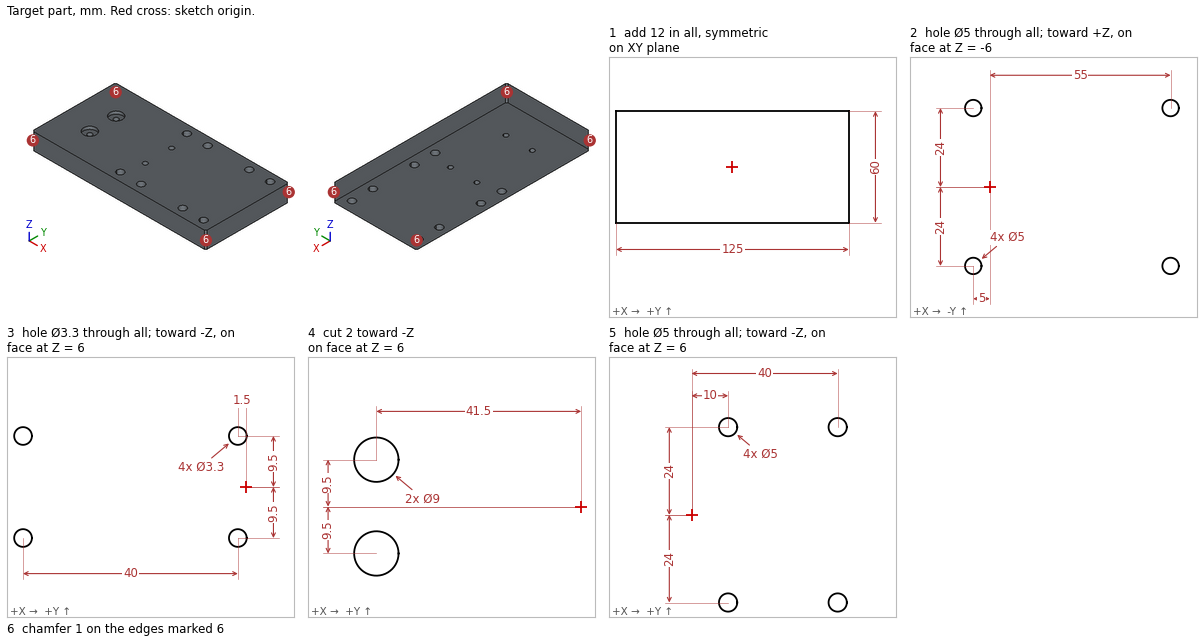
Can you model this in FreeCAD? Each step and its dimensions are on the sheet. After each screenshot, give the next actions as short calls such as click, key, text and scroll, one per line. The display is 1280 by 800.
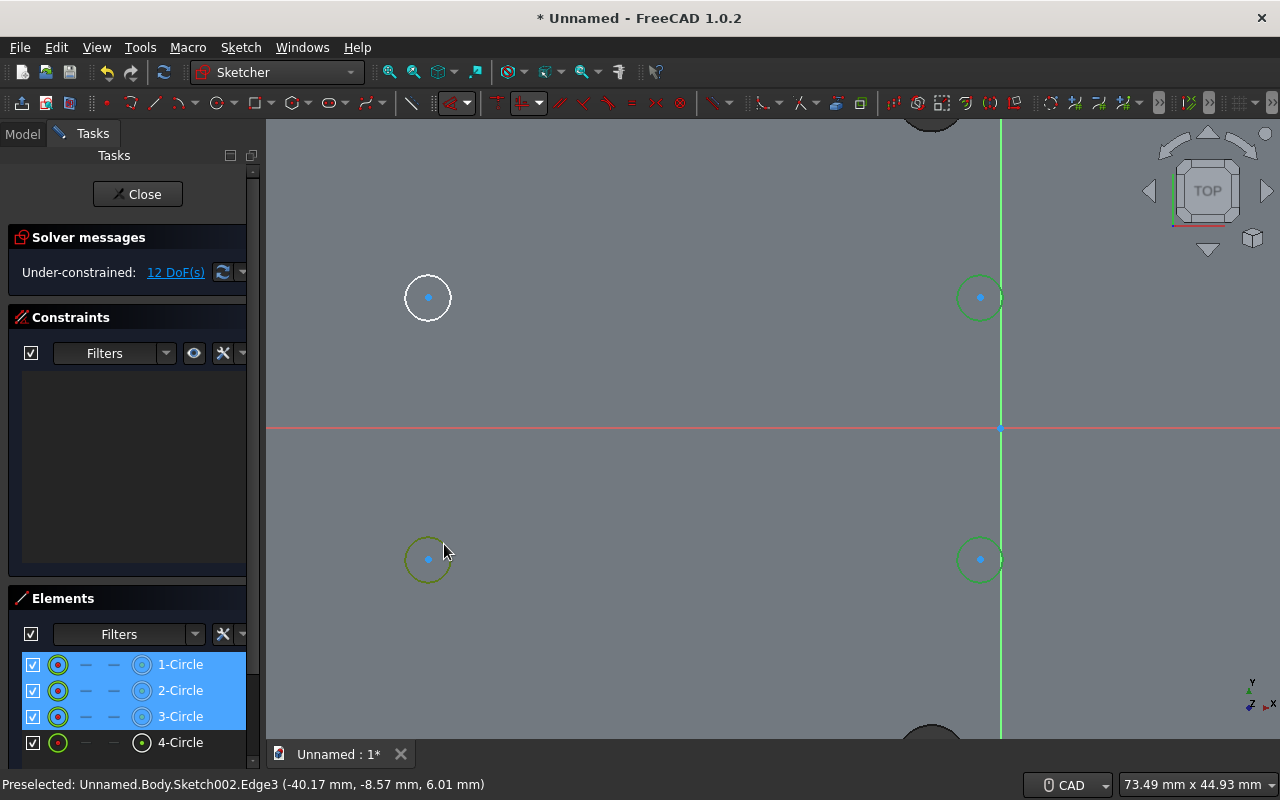
click(444, 282)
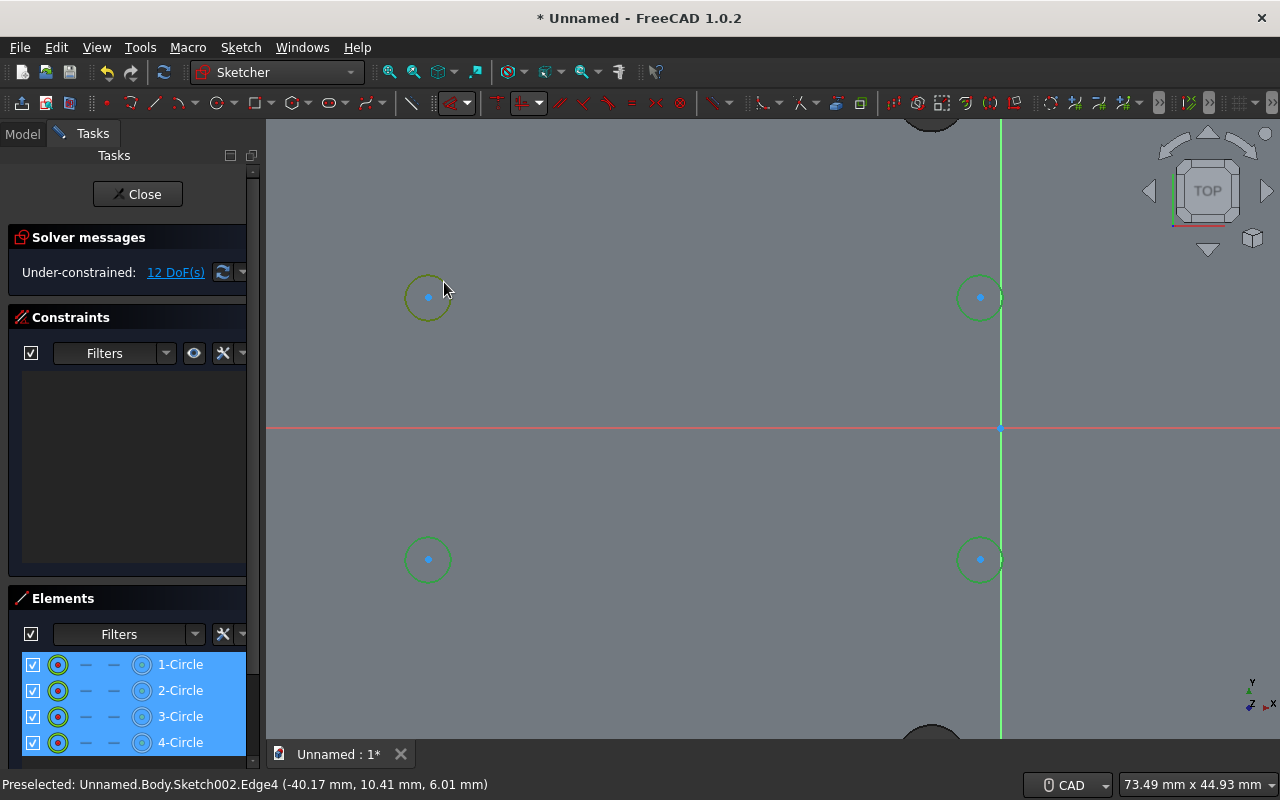
key(e)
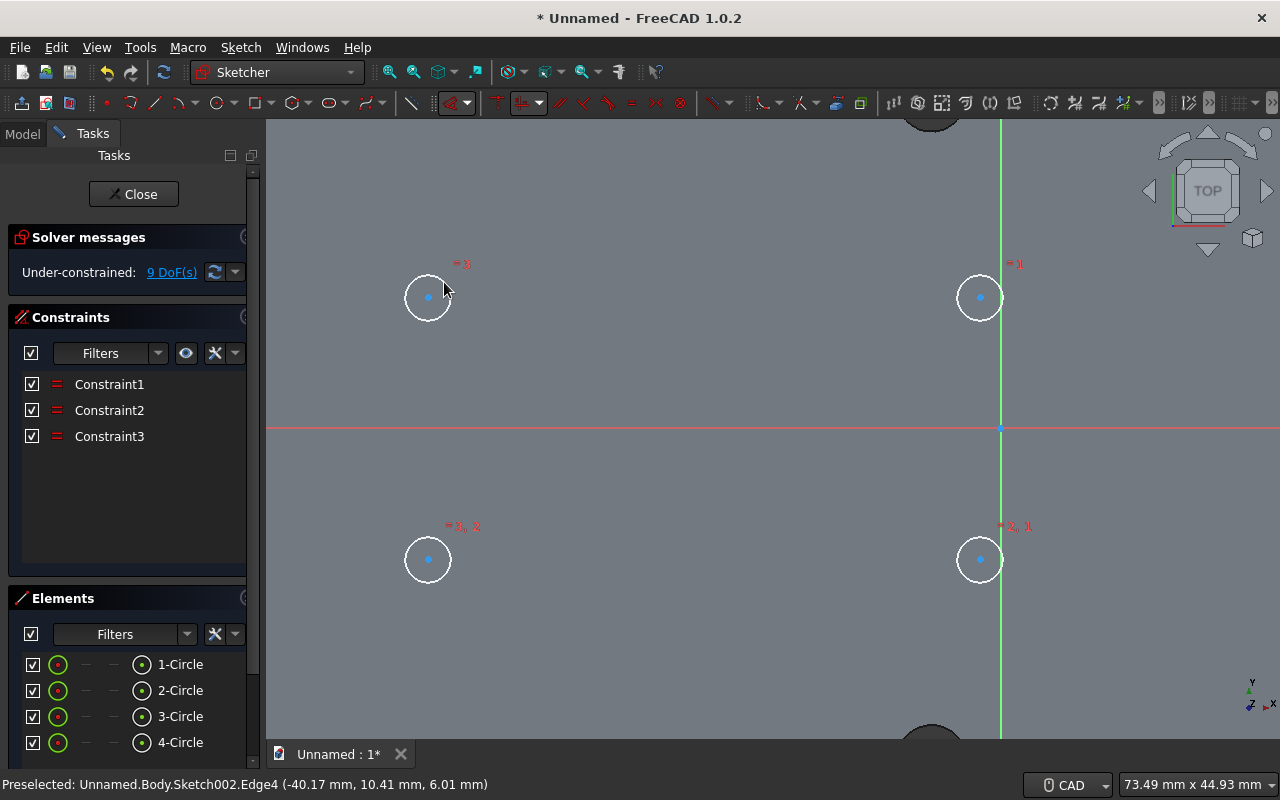
click(980, 298)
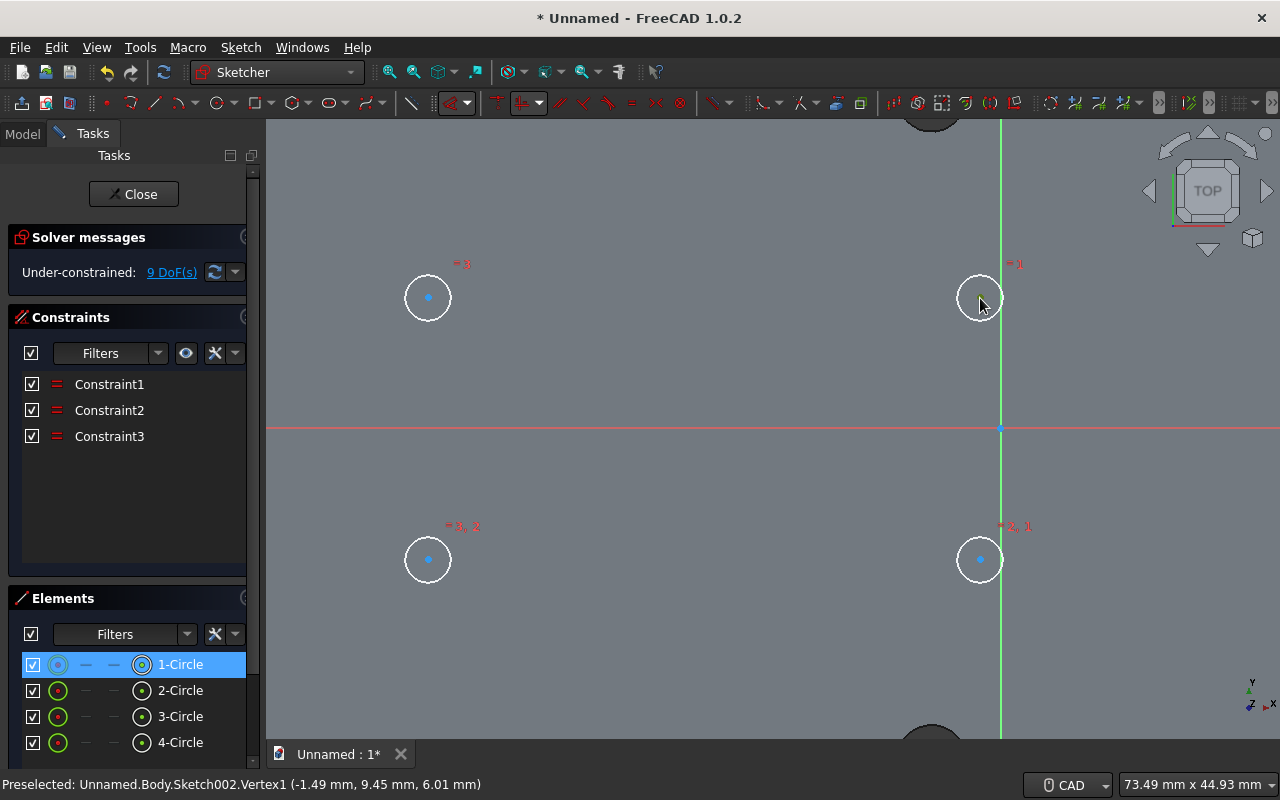
click(980, 560)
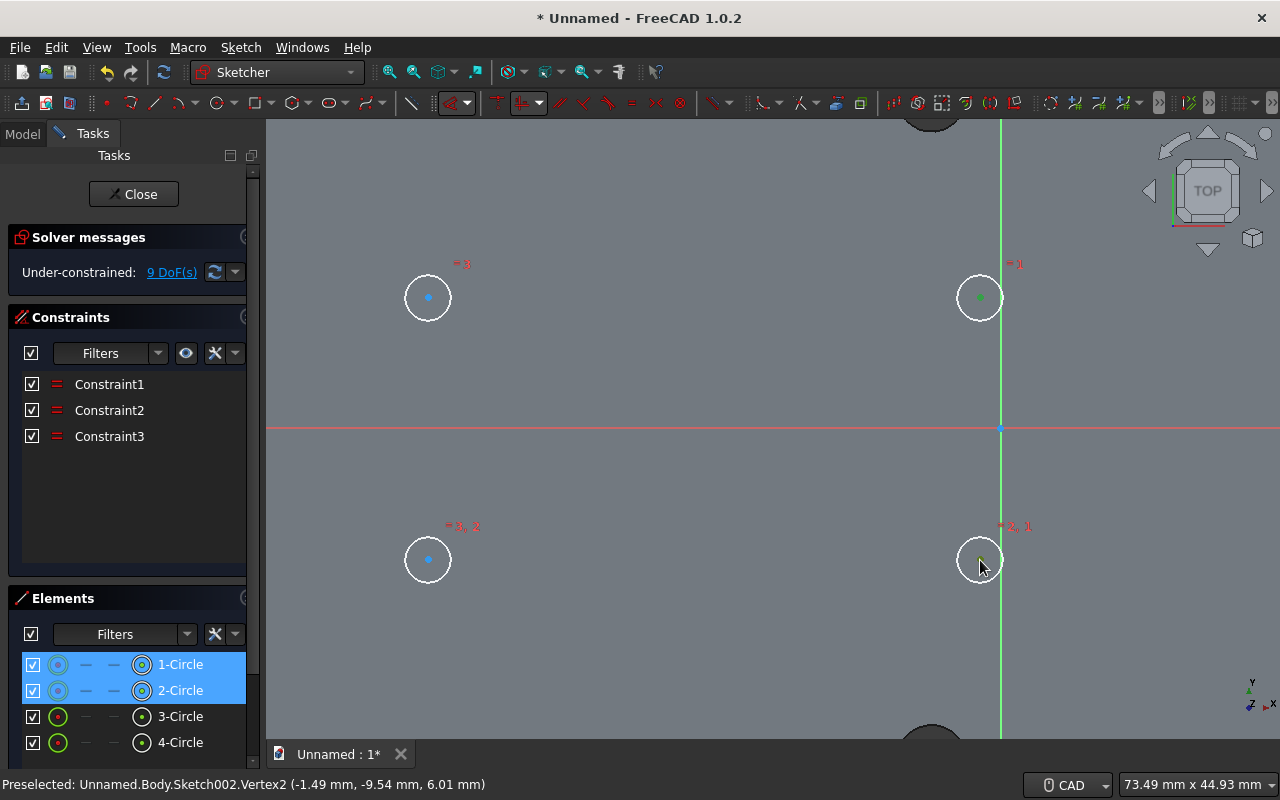
key(v)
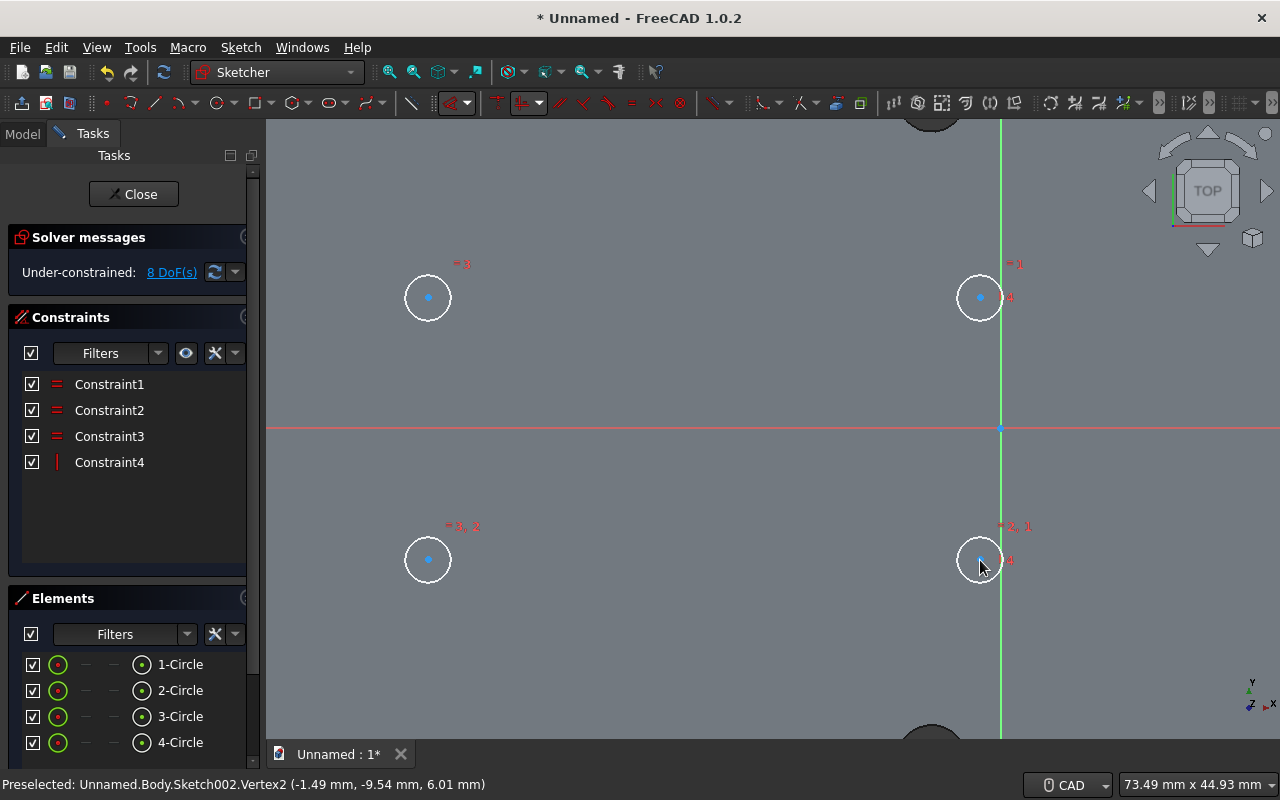
click(980, 560)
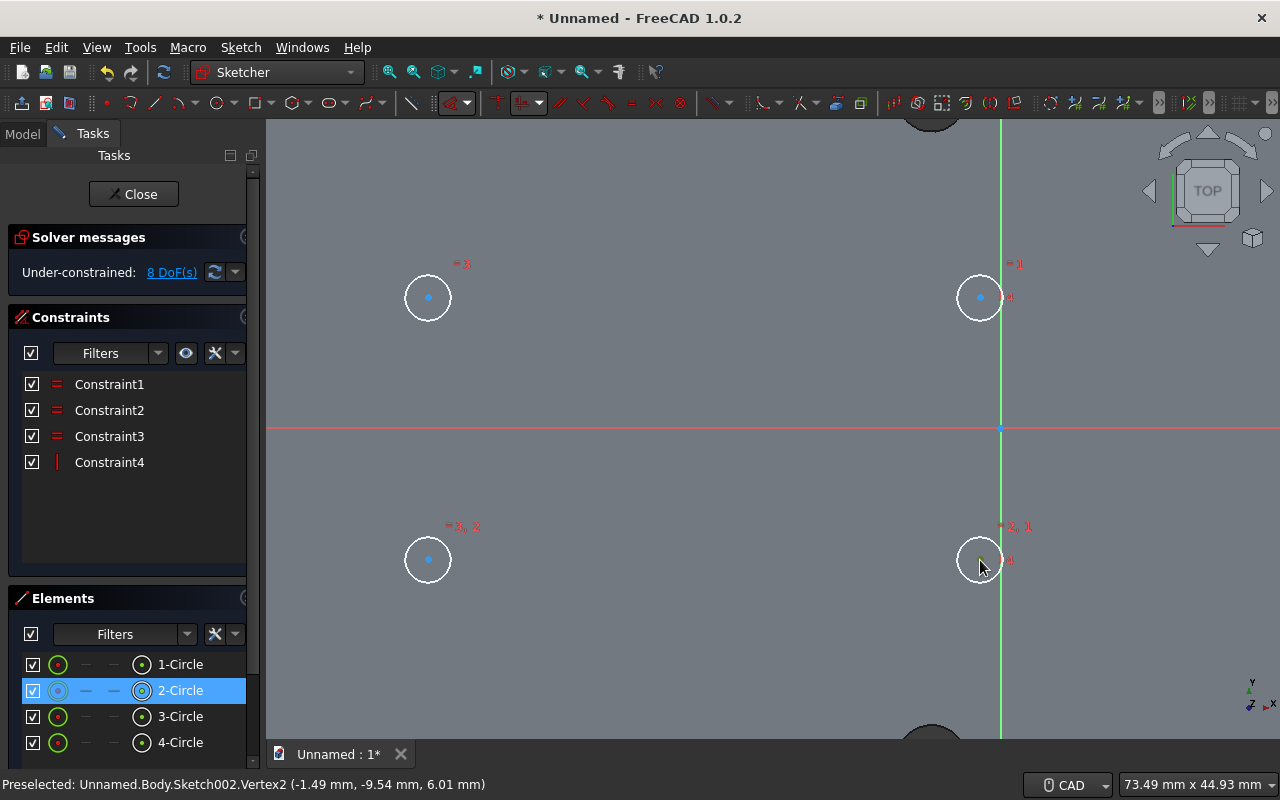
click(428, 560)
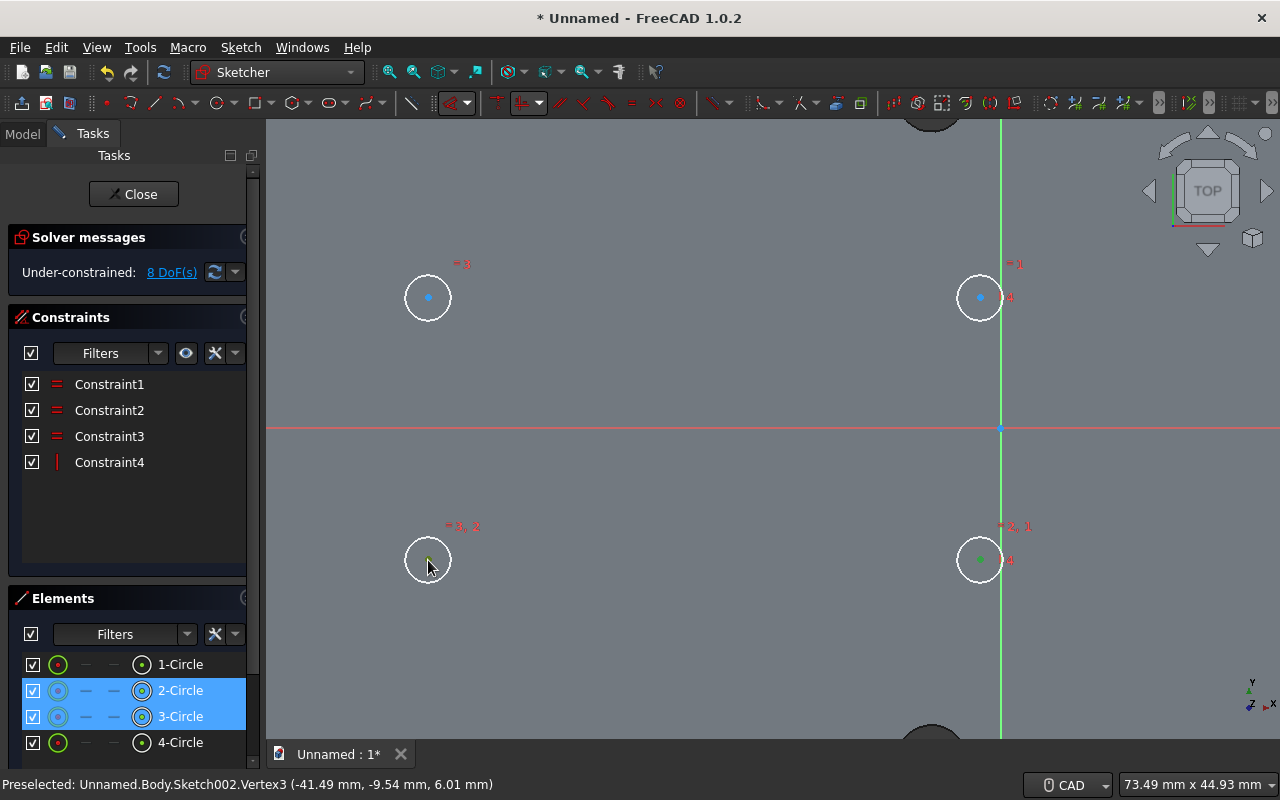
key(h)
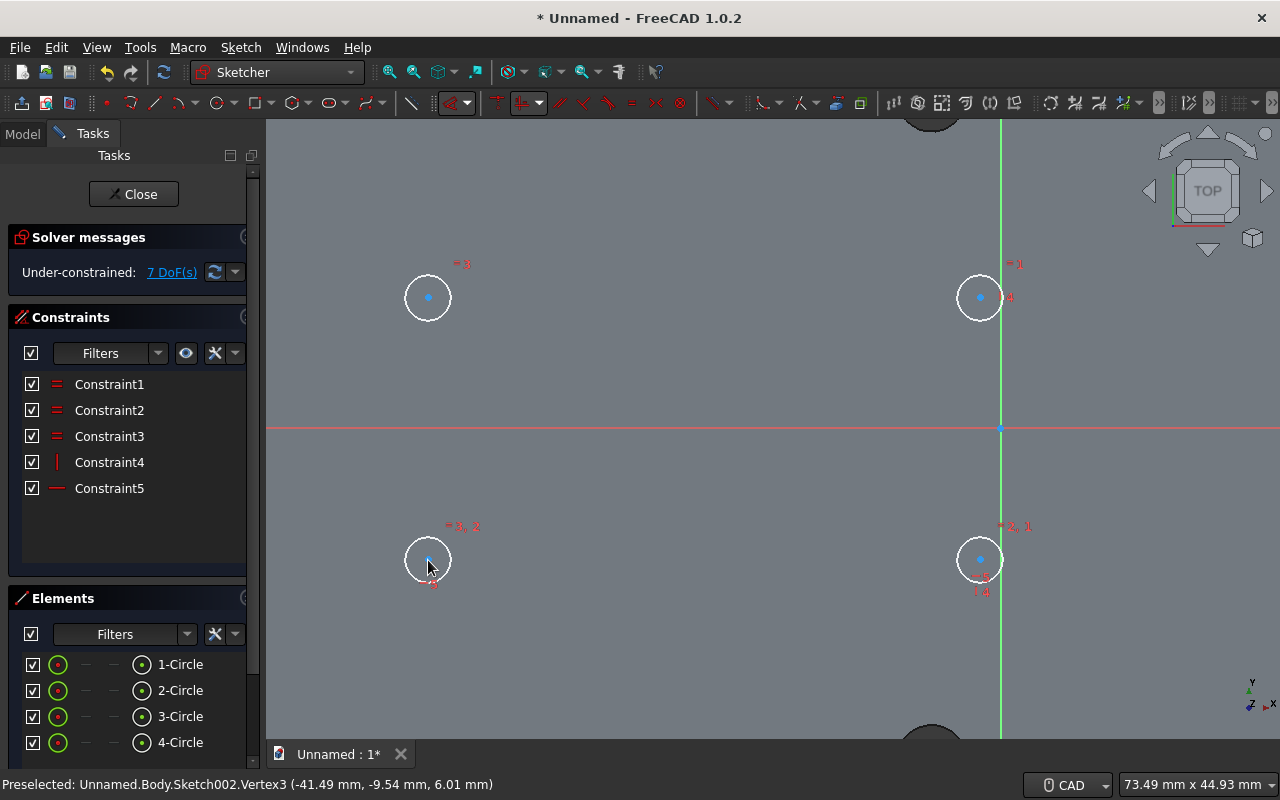
click(428, 560)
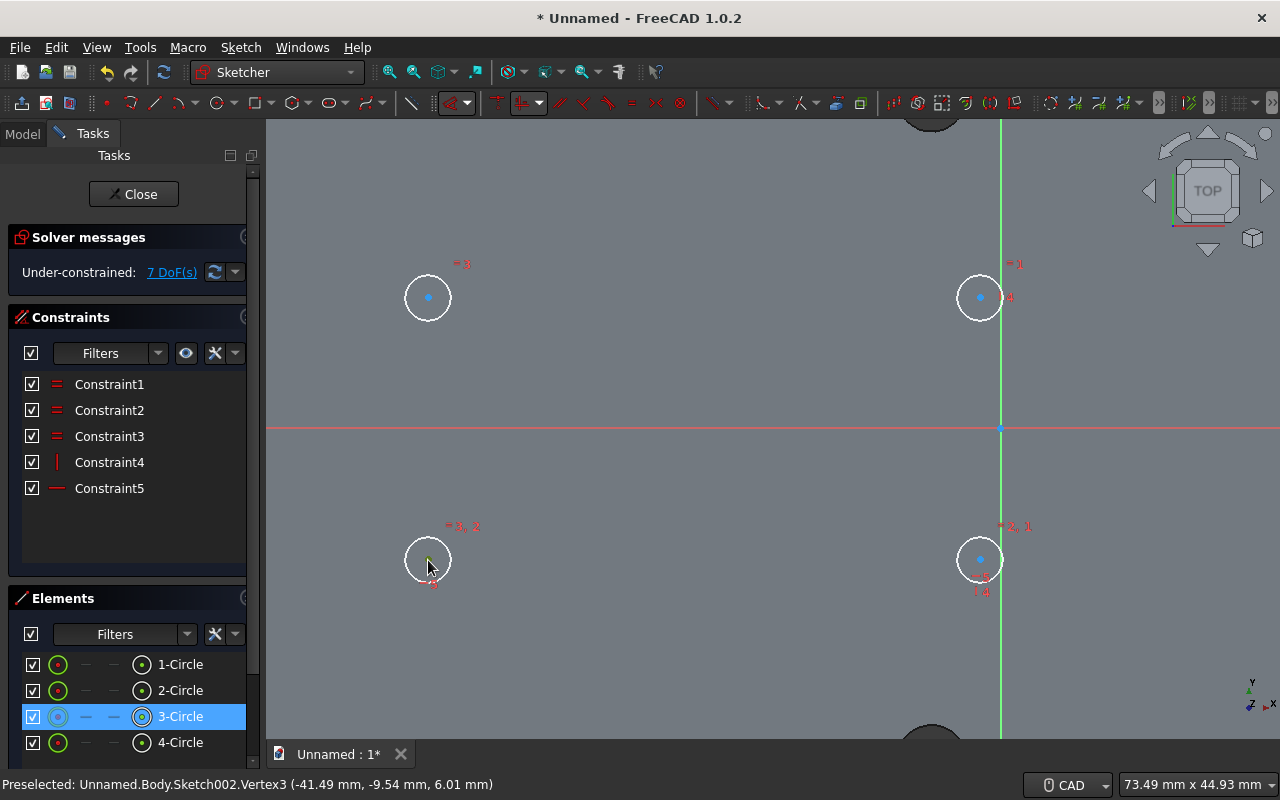
click(428, 298)